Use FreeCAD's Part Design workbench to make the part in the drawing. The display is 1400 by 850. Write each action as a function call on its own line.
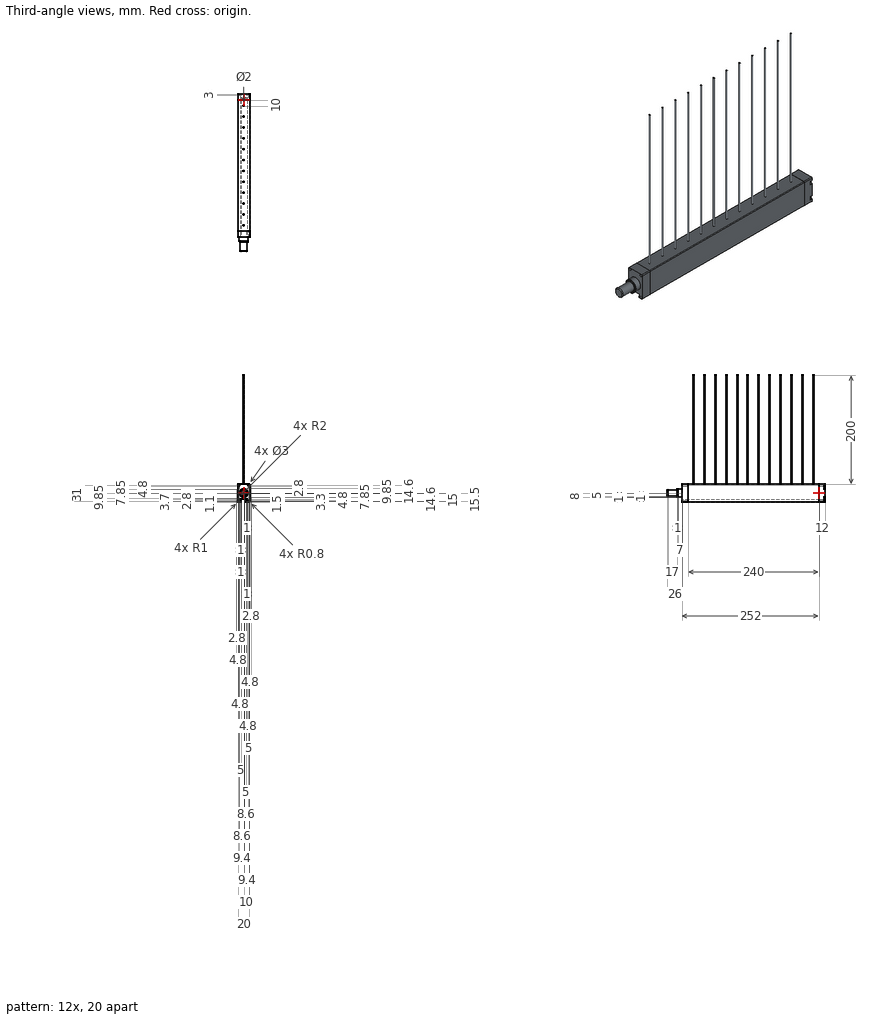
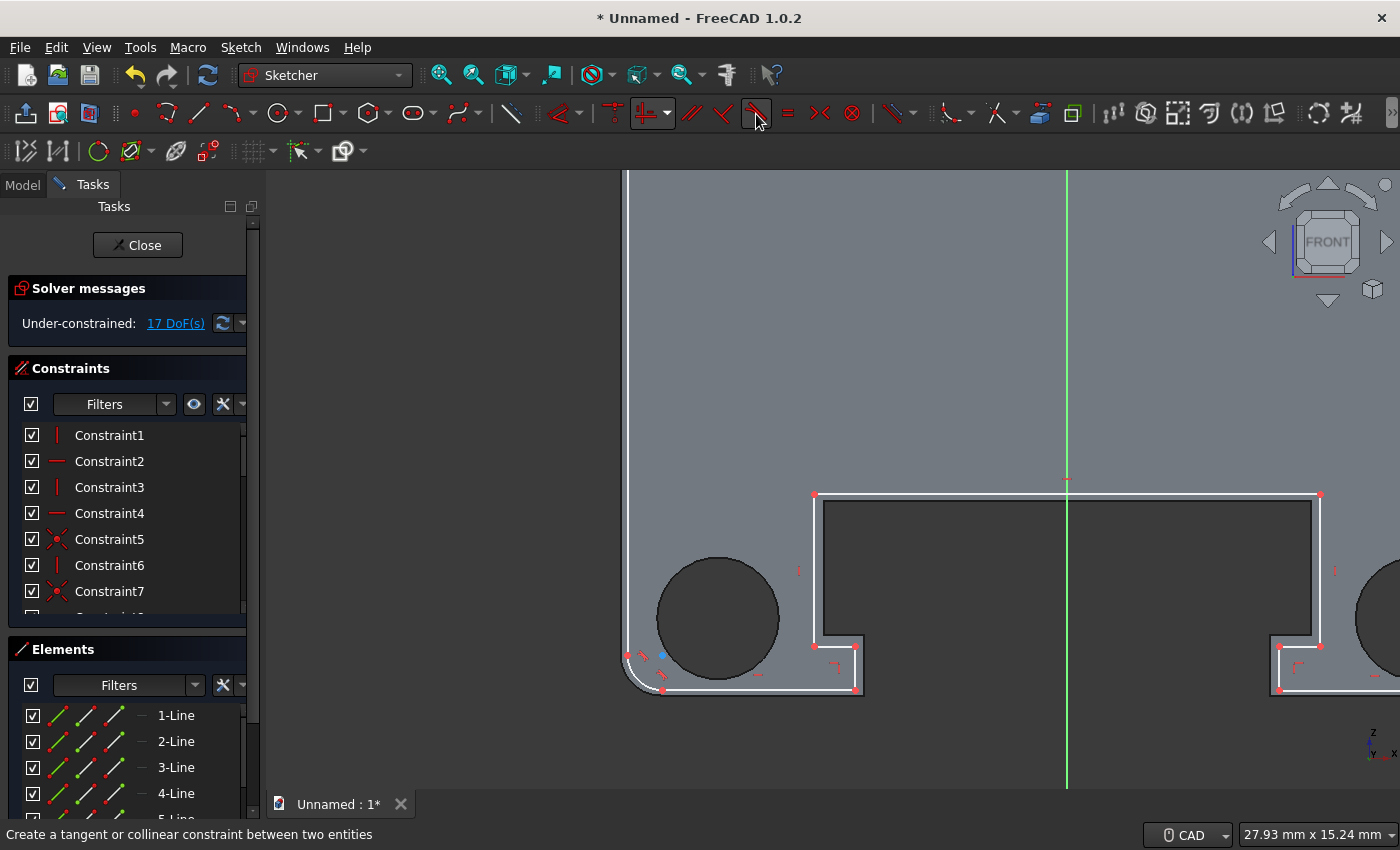
scroll(634, 675, down, 6)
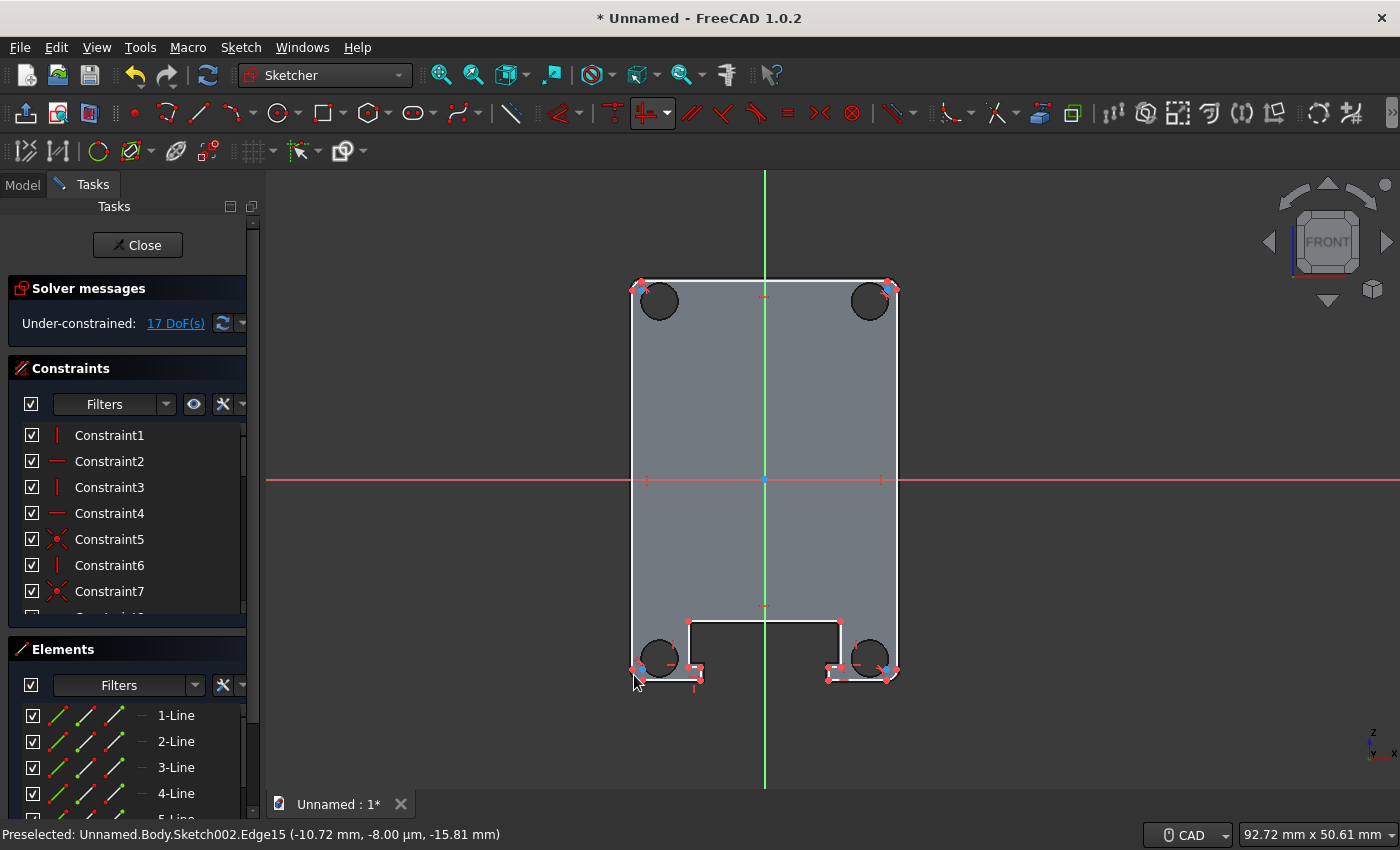
click(869, 680)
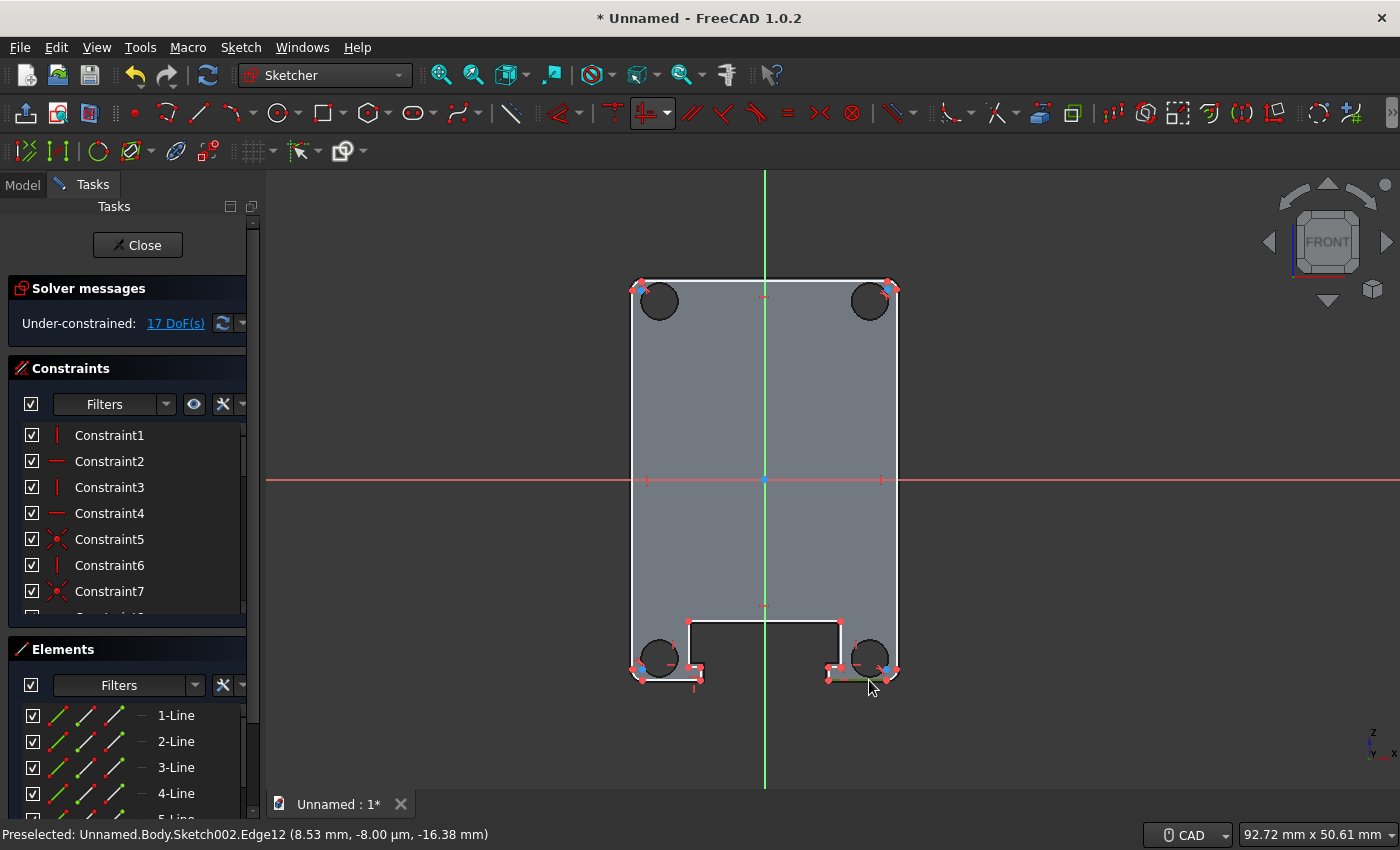
scroll(894, 677, up, 3)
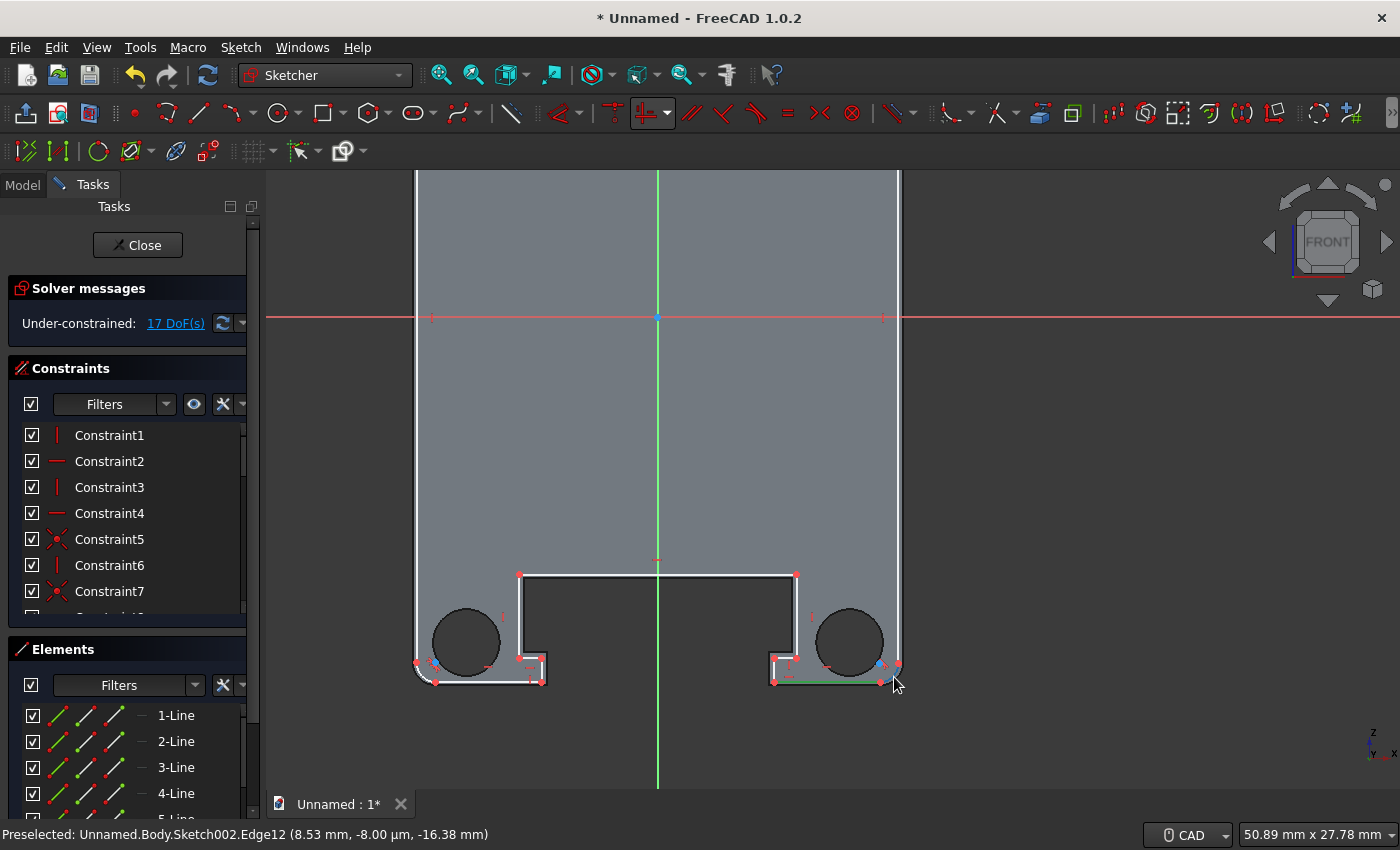
click(893, 676)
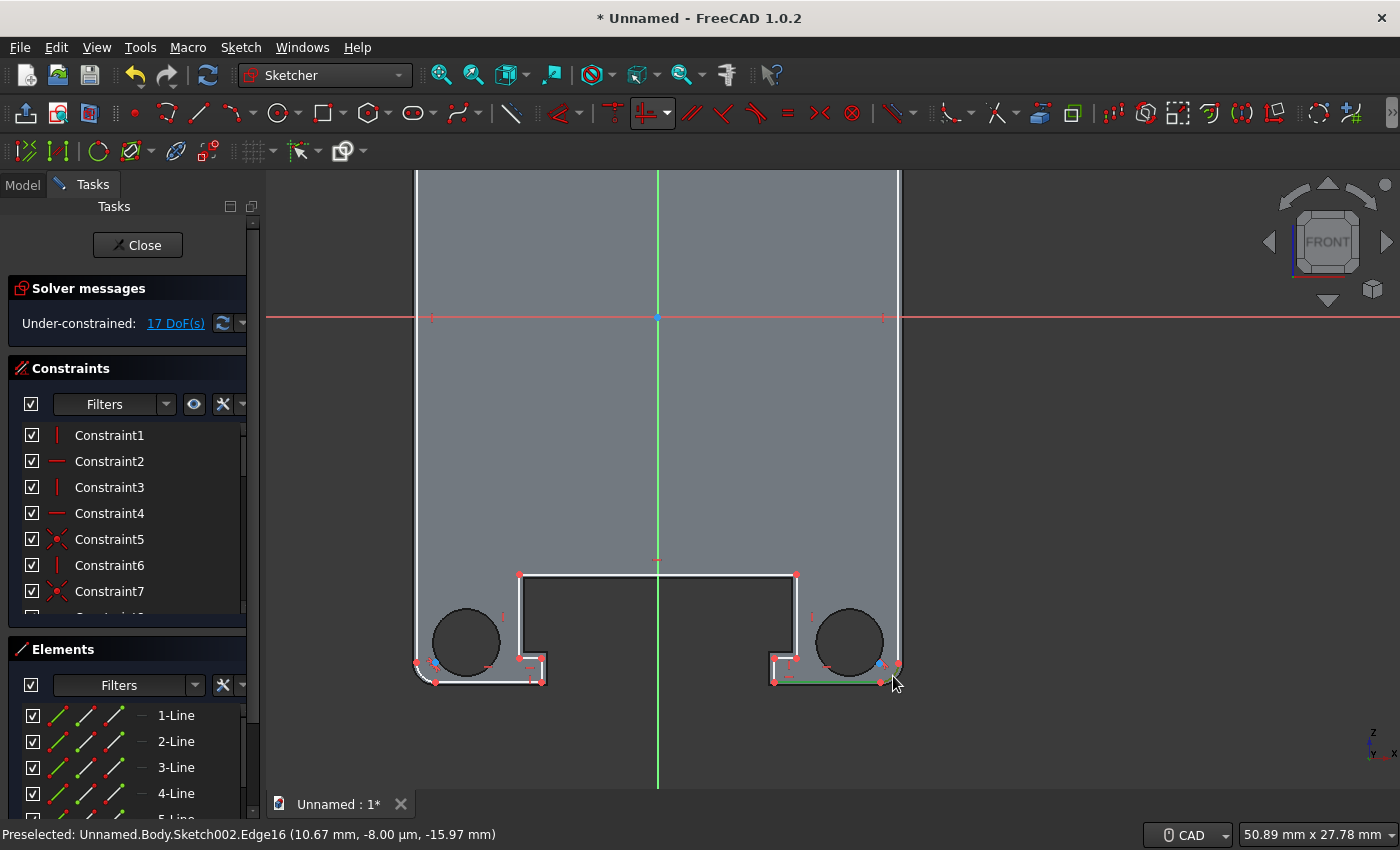
key(t)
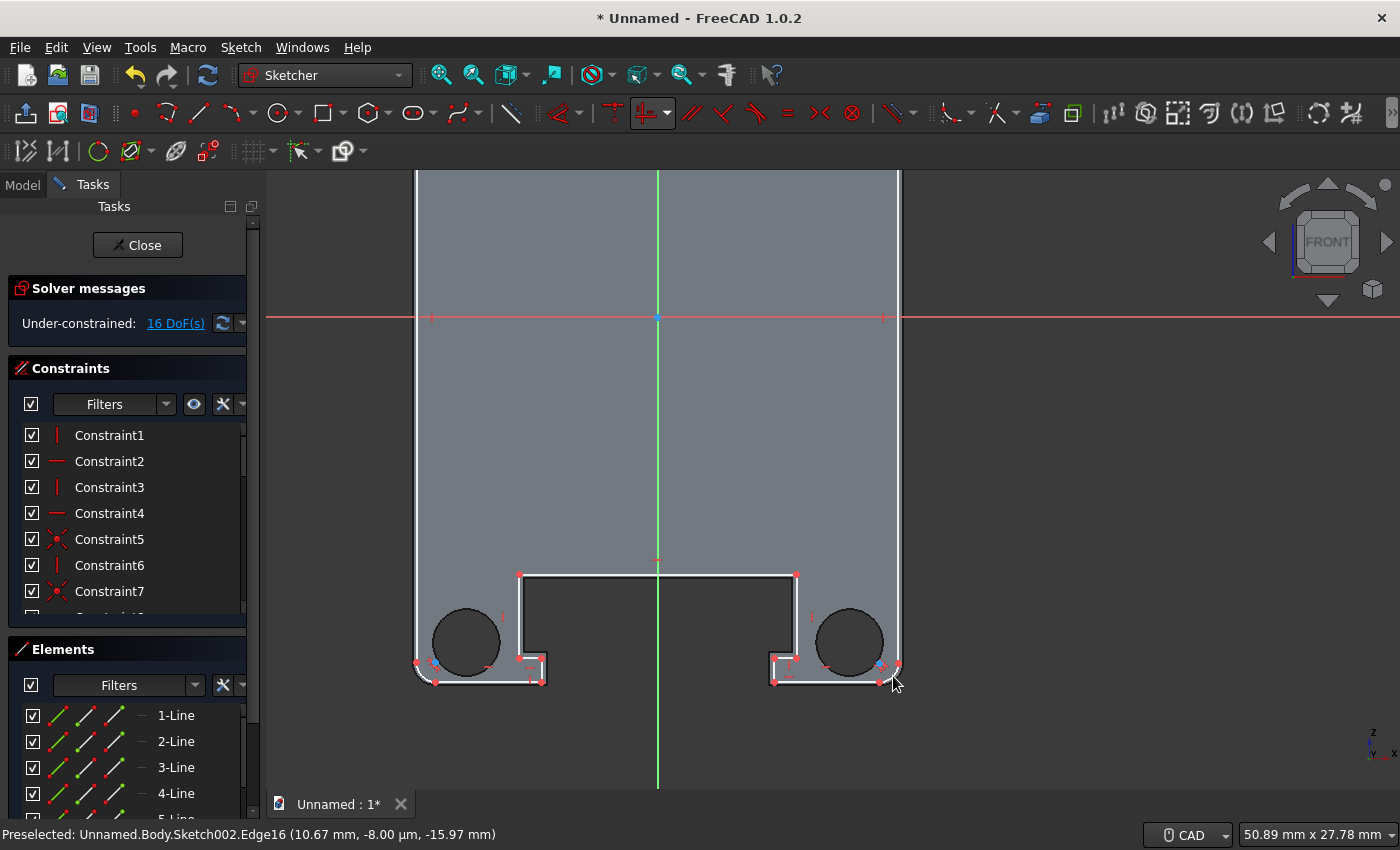
scroll(894, 677, down, 3)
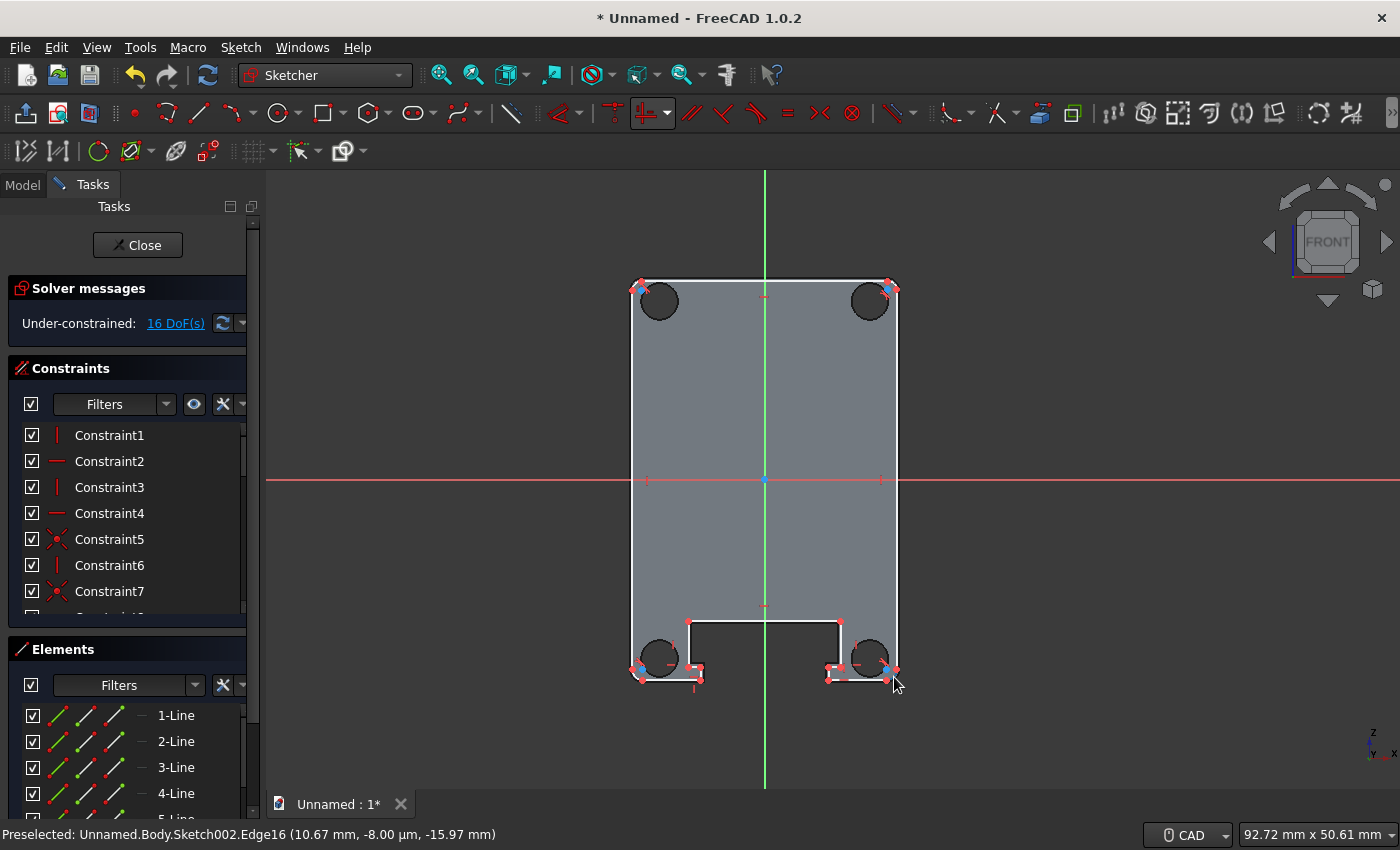
scroll(894, 284, up, 4)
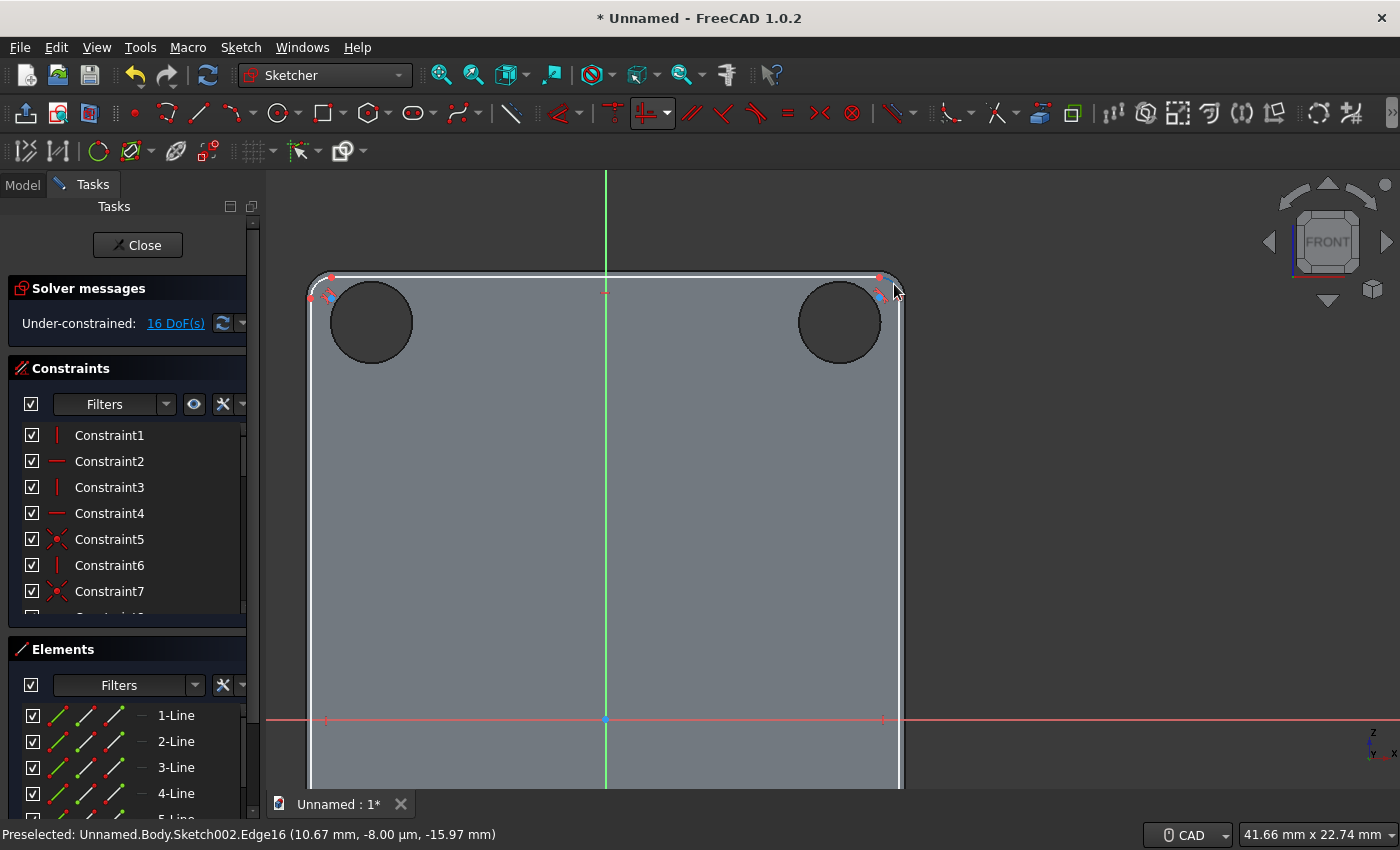
click(894, 283)